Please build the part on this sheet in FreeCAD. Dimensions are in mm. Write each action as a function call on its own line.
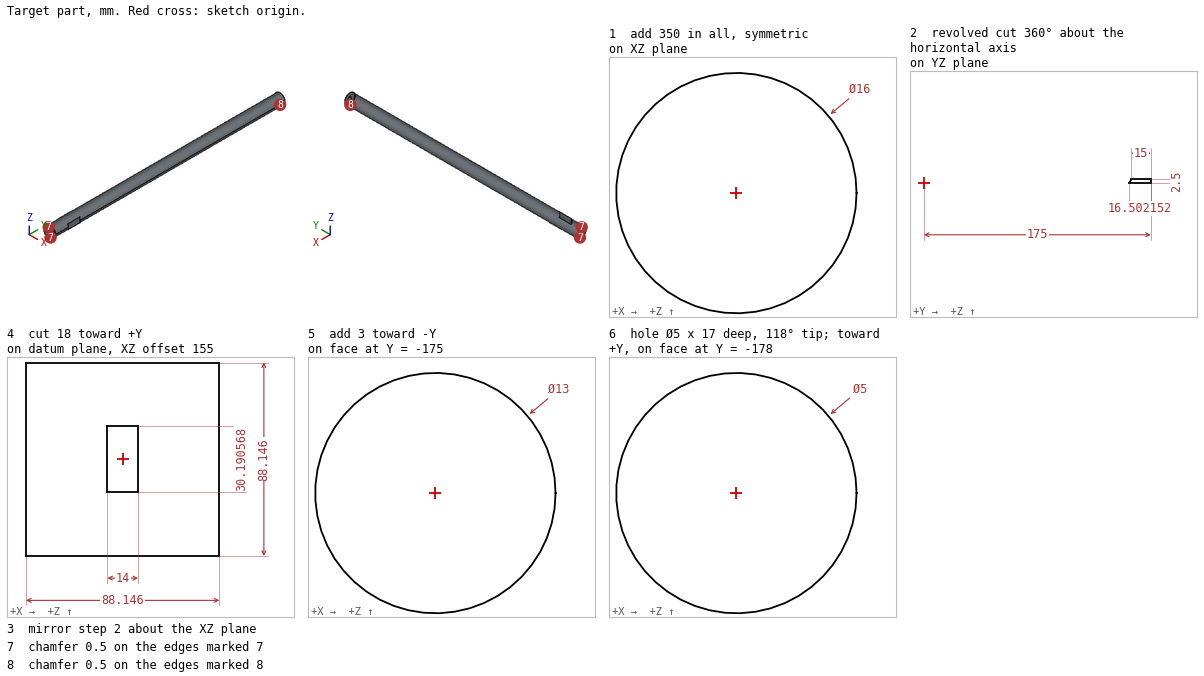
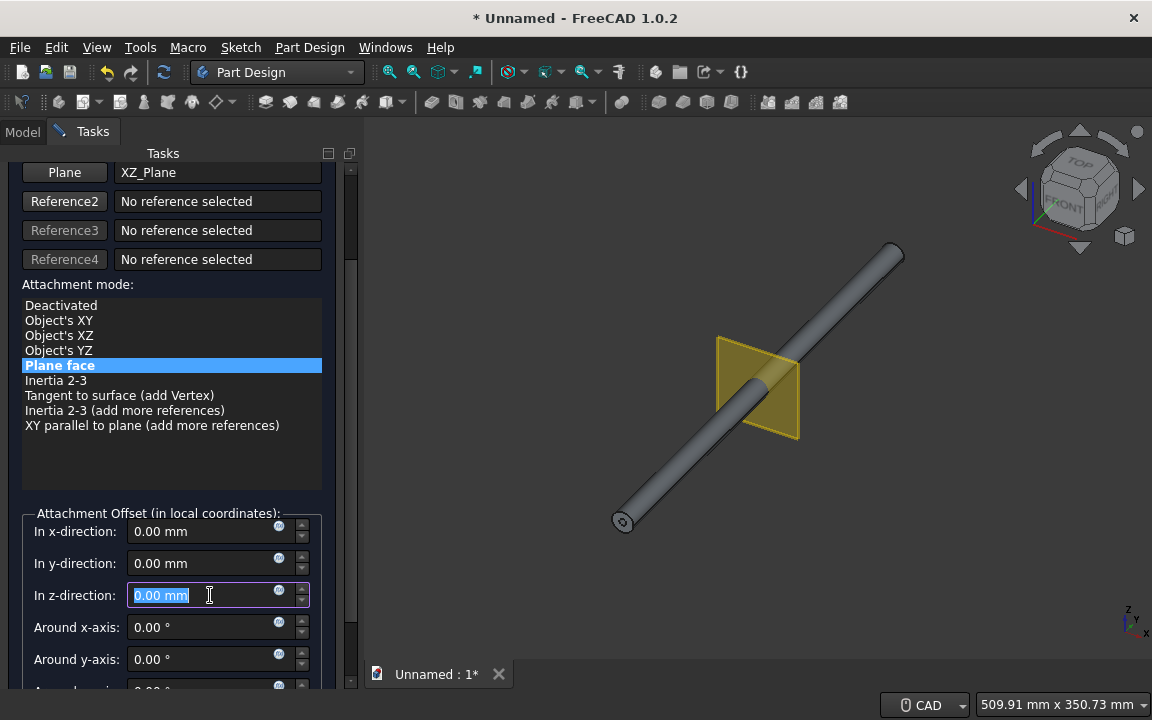
text(155)
key(Tab)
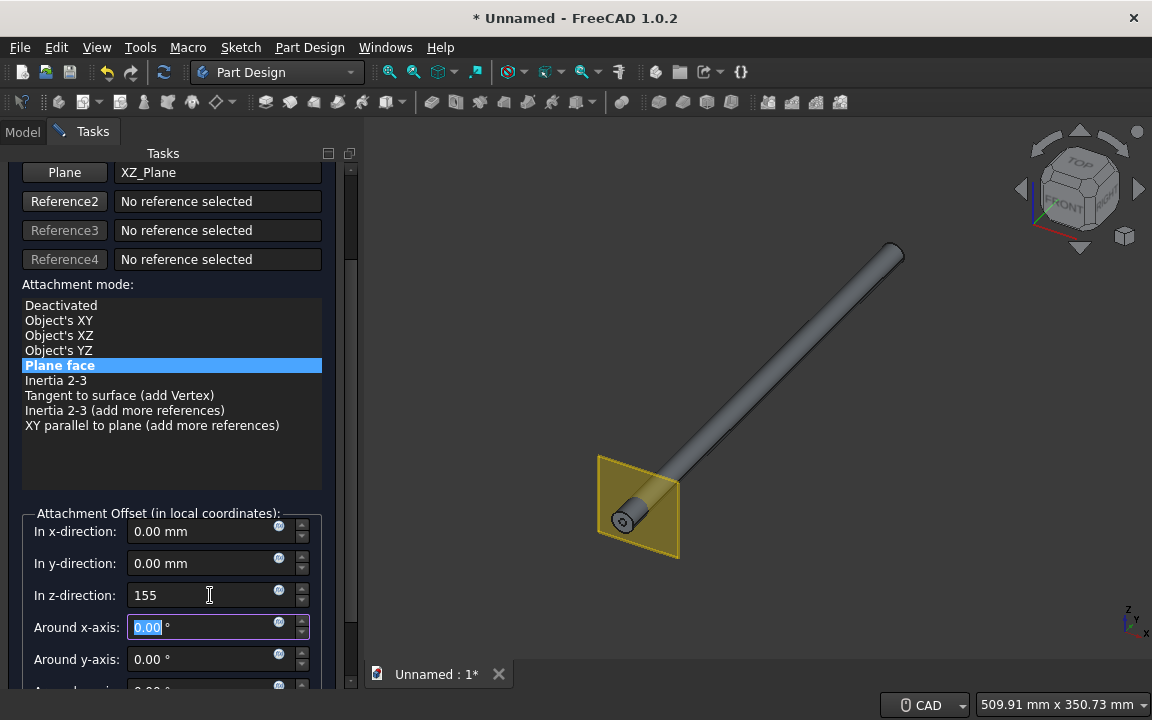
scroll(351, 426, up, 3)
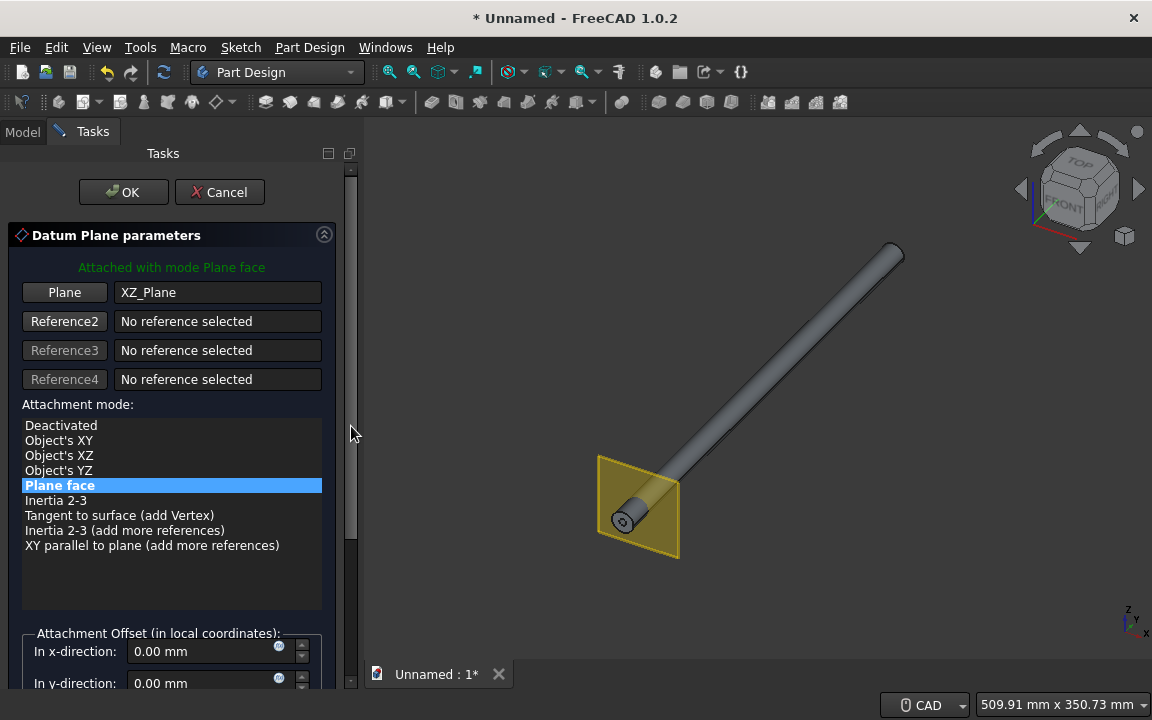
click(124, 192)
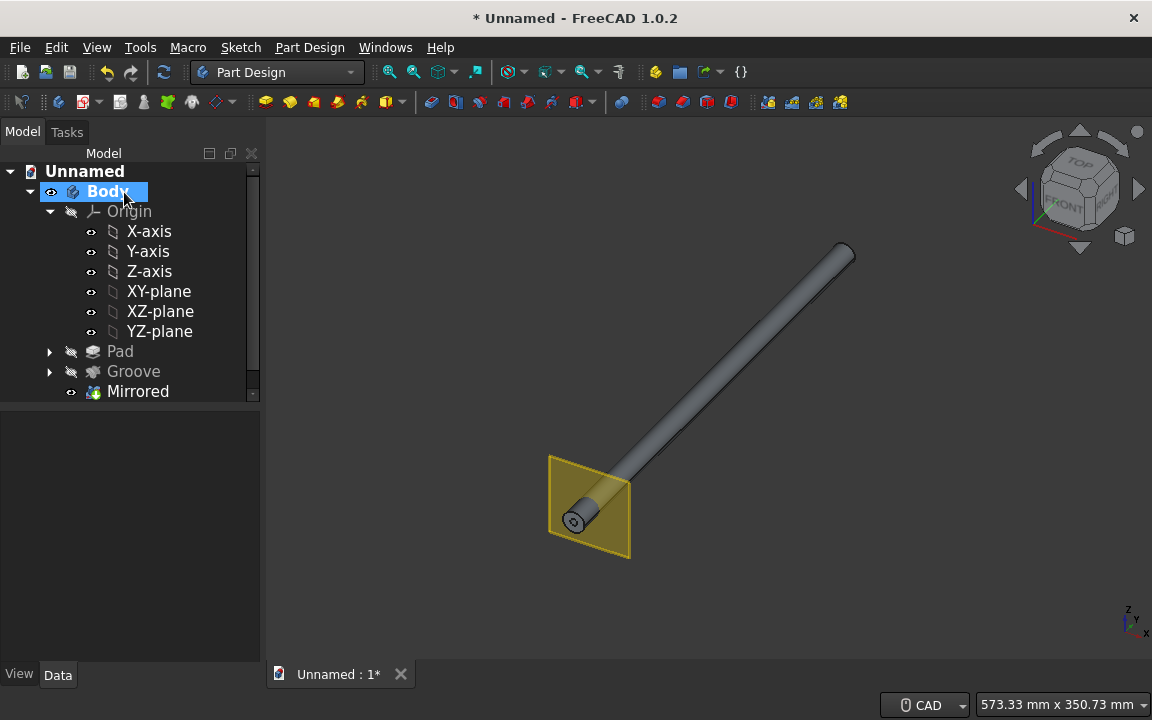
scroll(100, 287, down, 3)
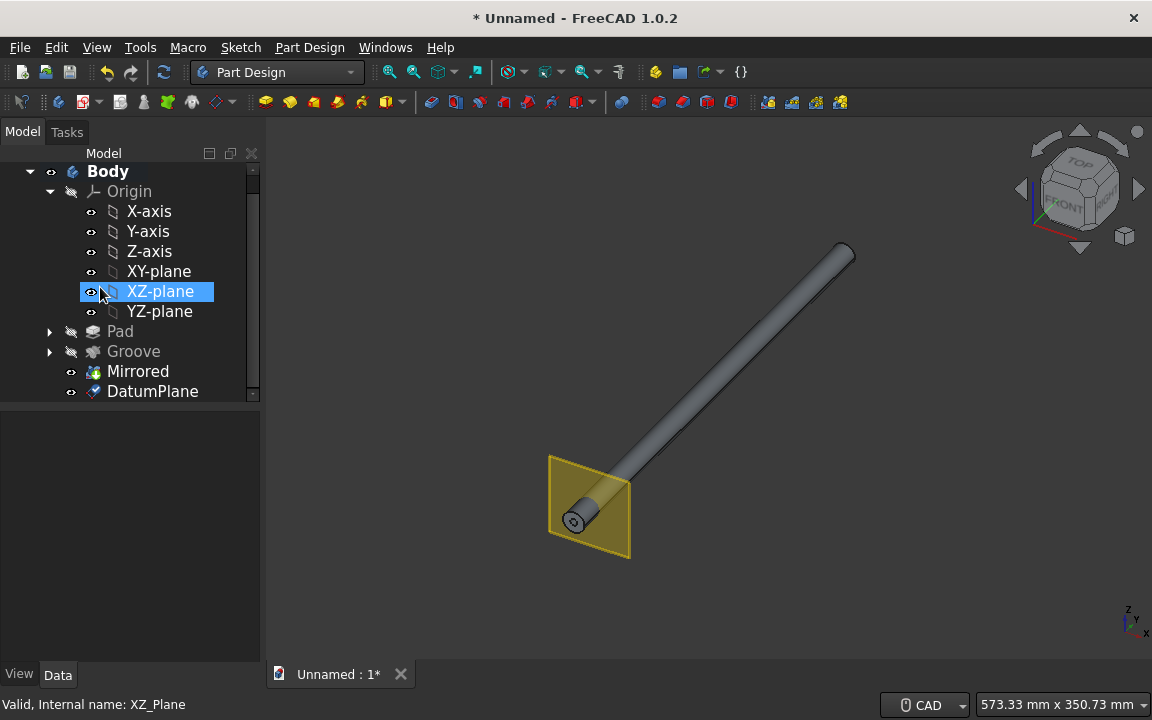
click(116, 392)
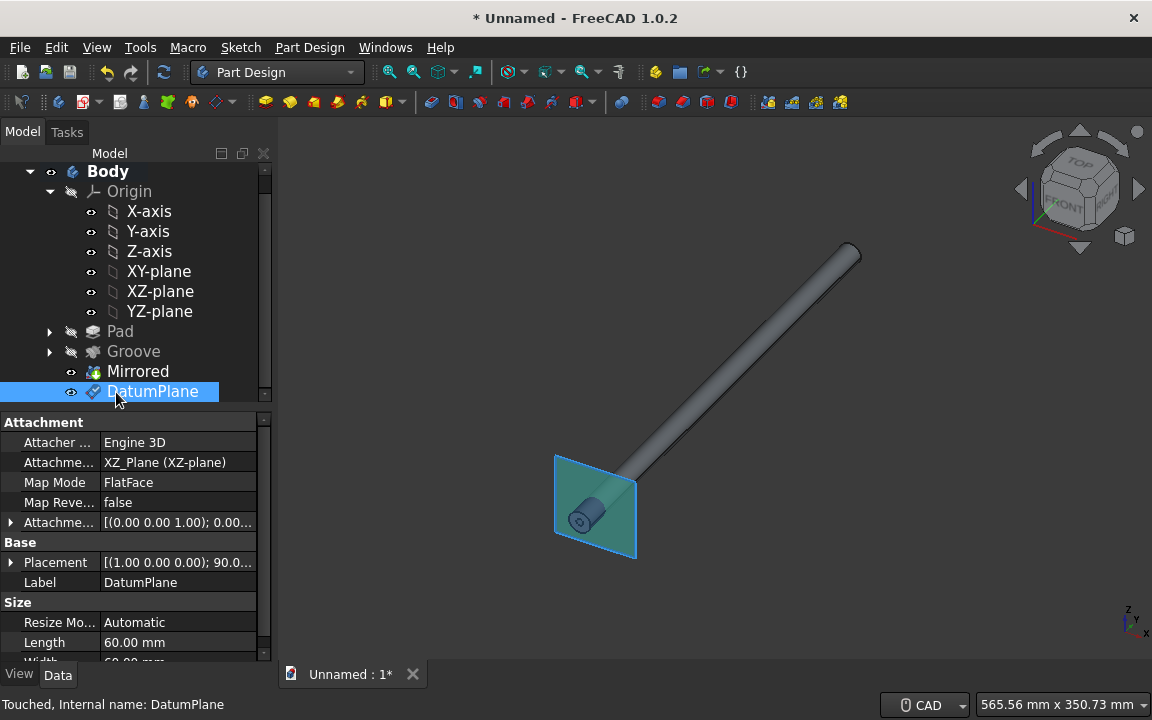
click(84, 102)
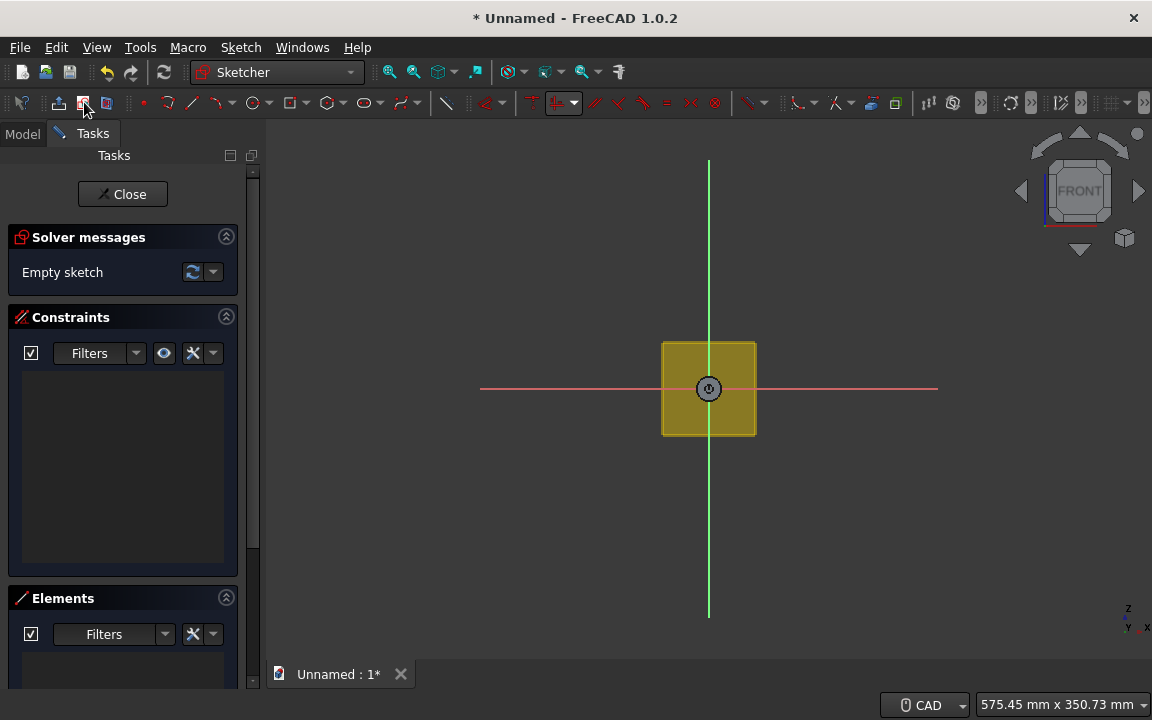
key(q)
key(s)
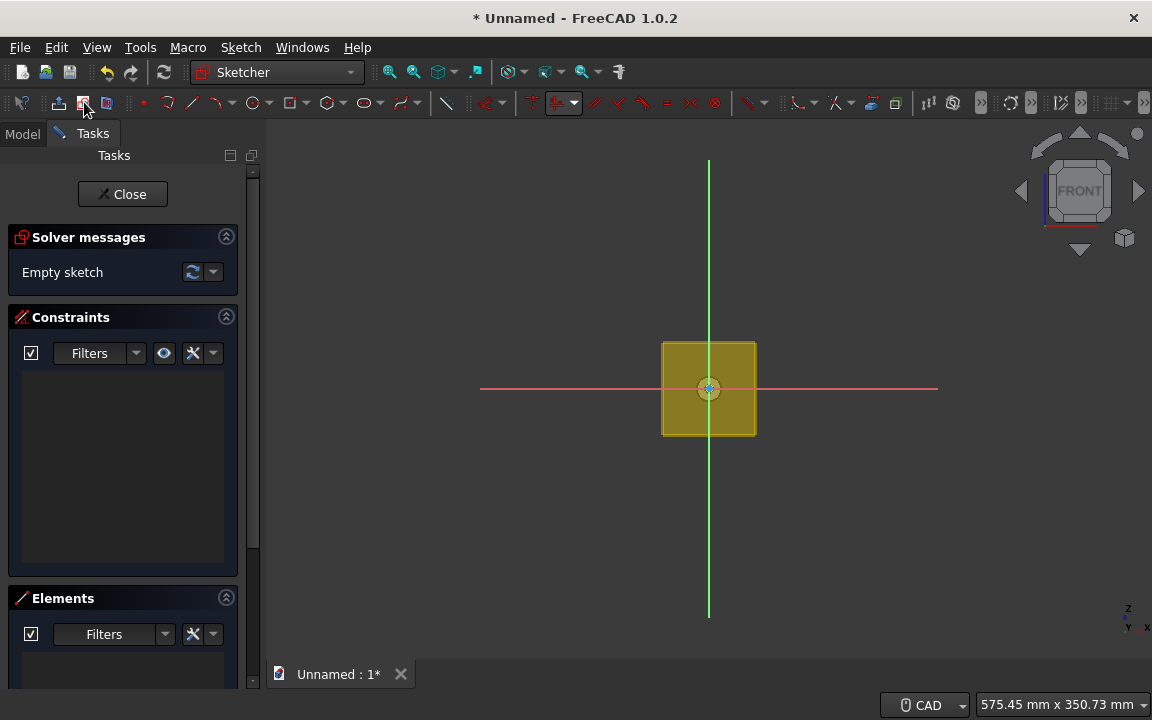
scroll(749, 389, up, 5)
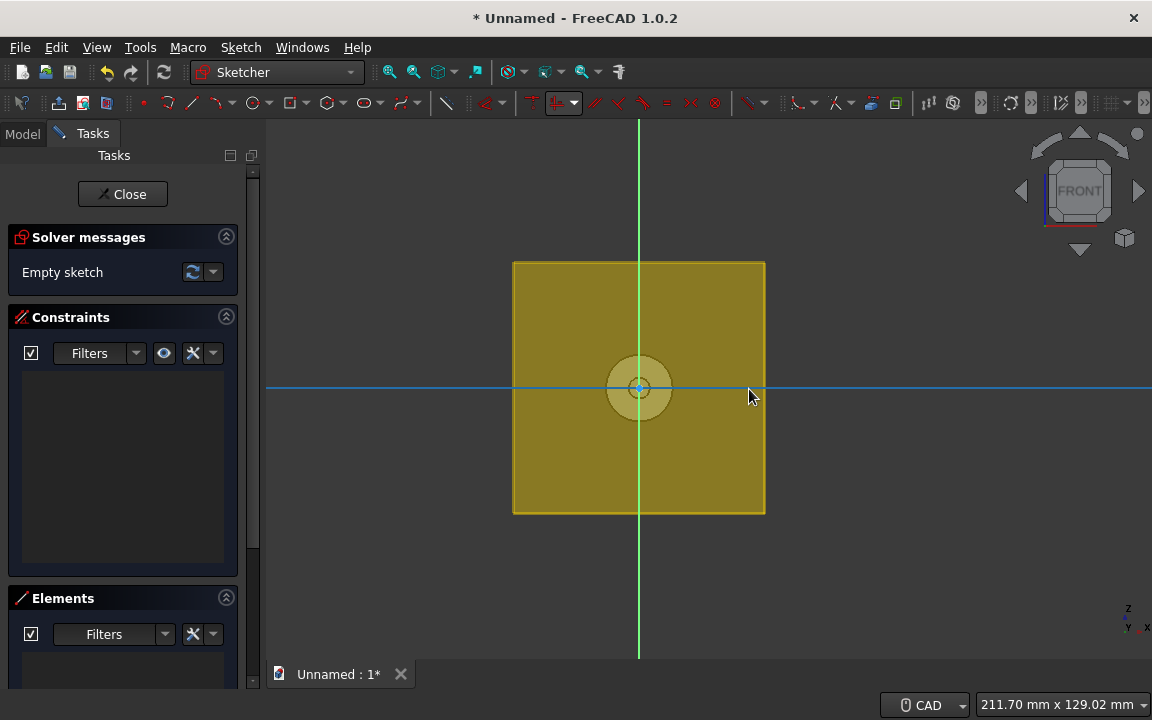
key(g)
key(v)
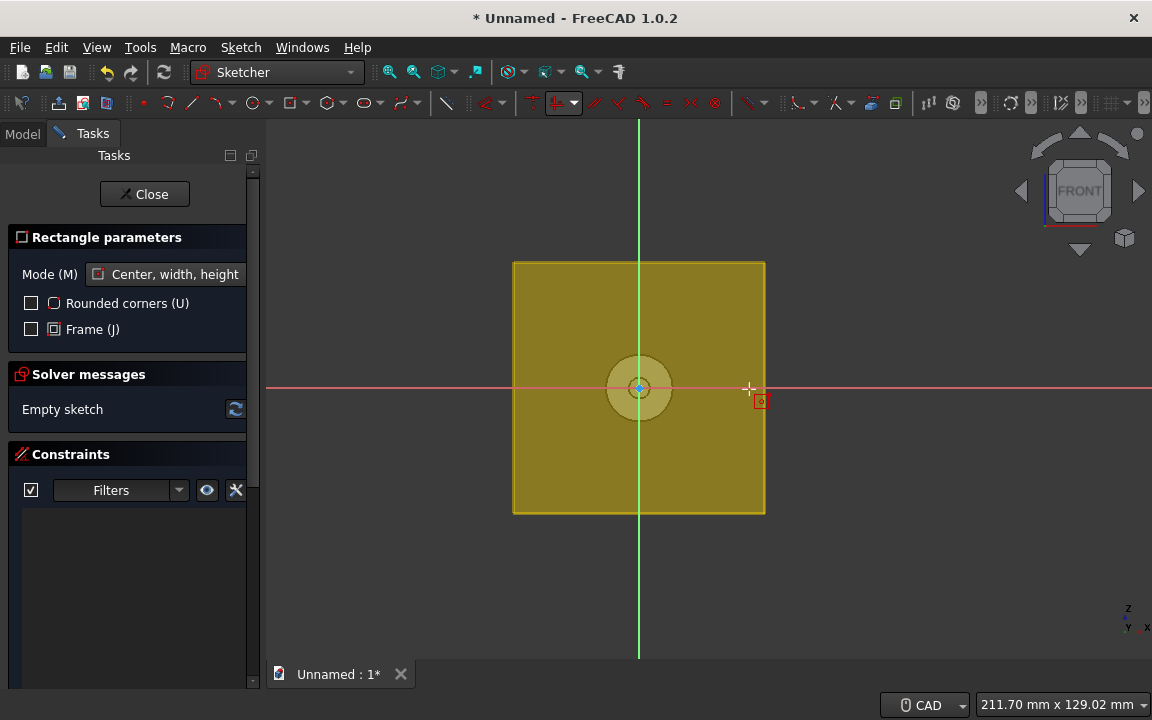
click(639, 388)
move(824, 204)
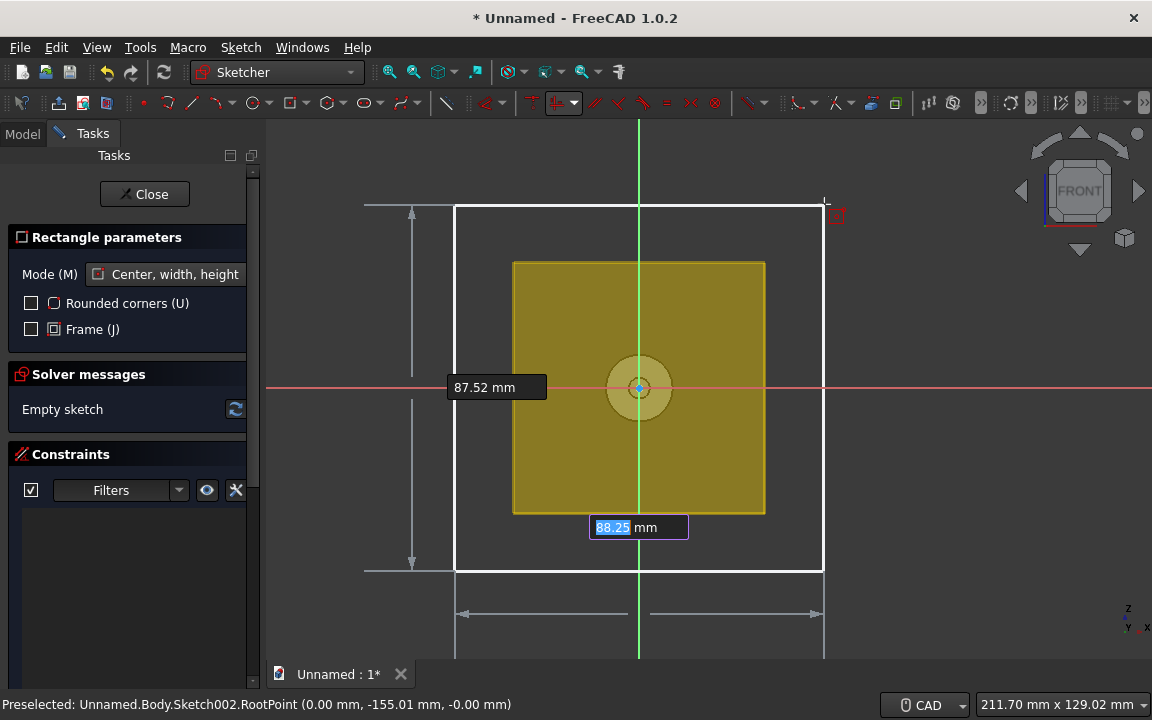
text(88.146)
key(Tab)
text(88.146)
key(Return)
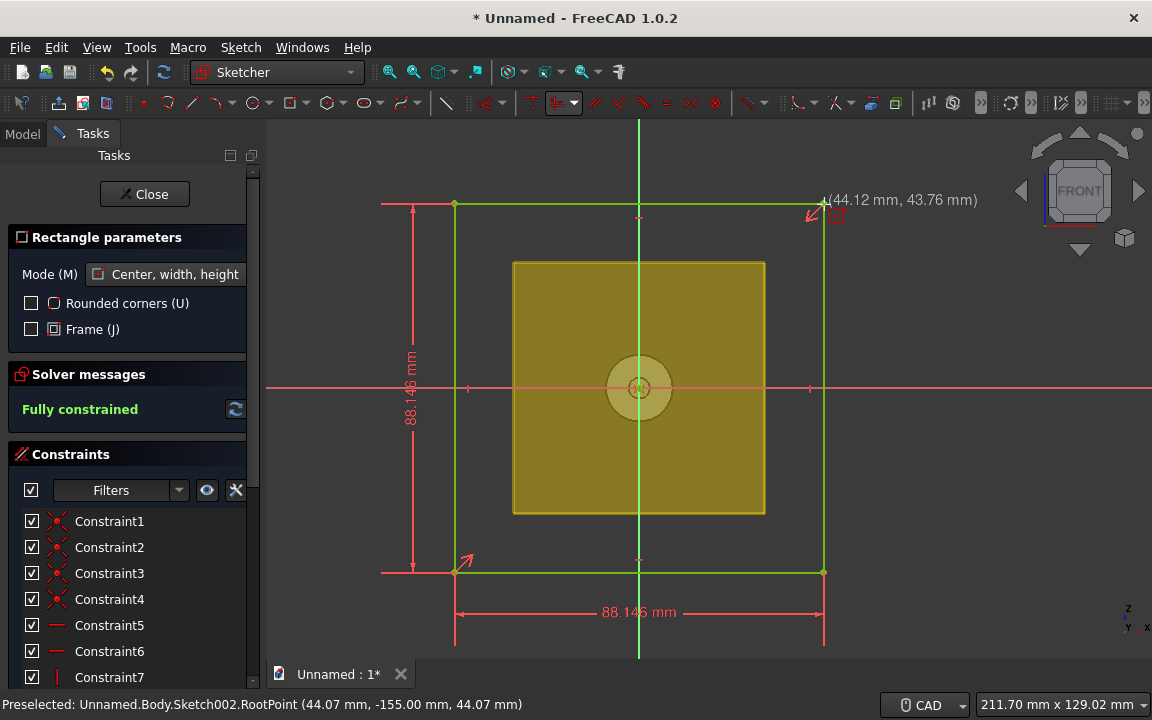
click(639, 388)
move(669, 325)